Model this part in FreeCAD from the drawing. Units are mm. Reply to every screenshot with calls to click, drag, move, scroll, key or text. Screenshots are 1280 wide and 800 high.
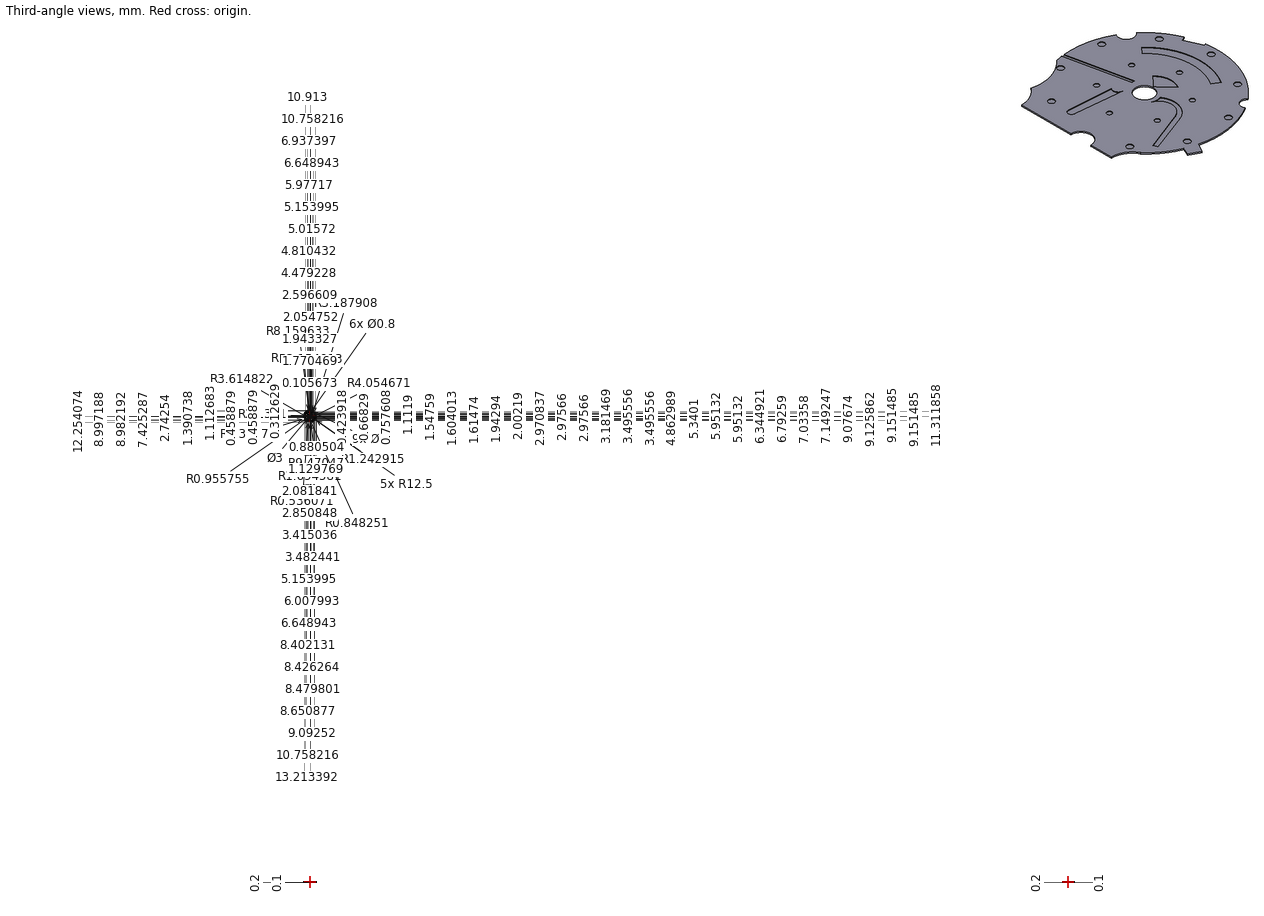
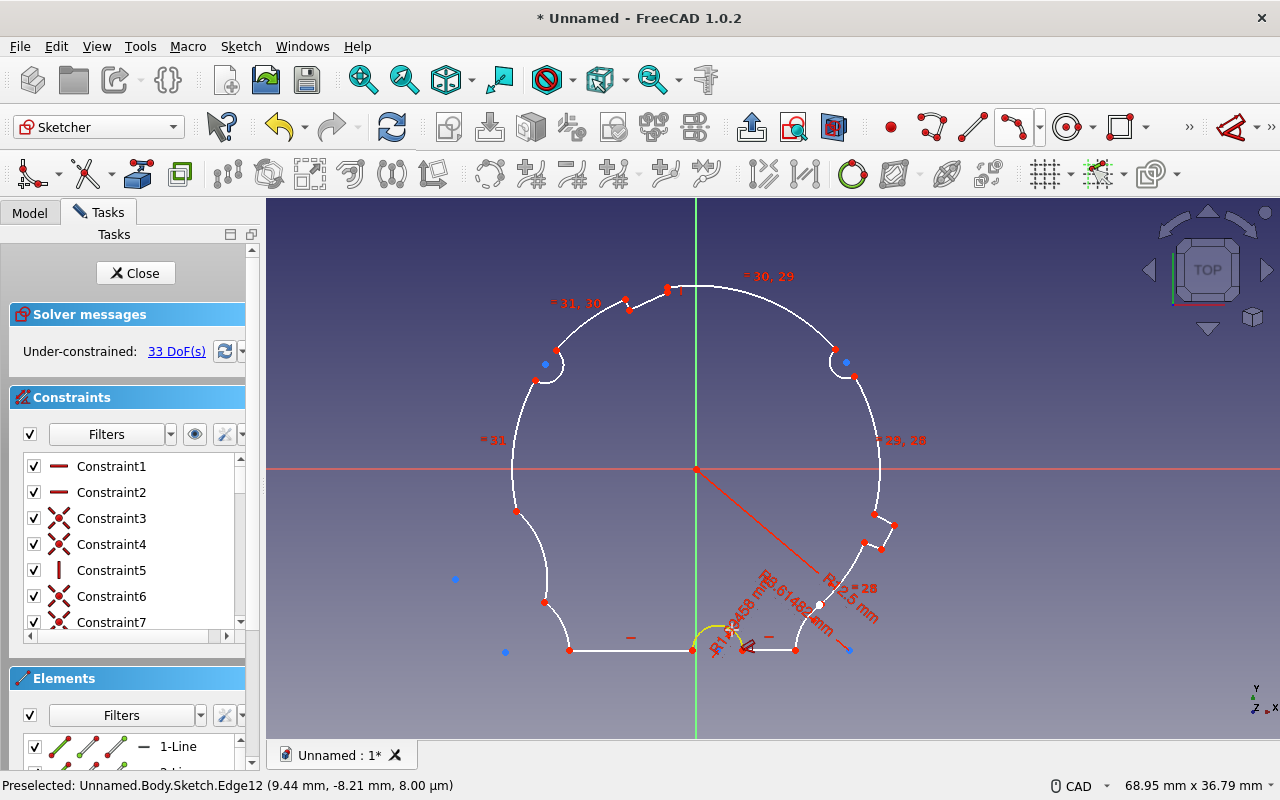
scroll(830, 362, up, 6)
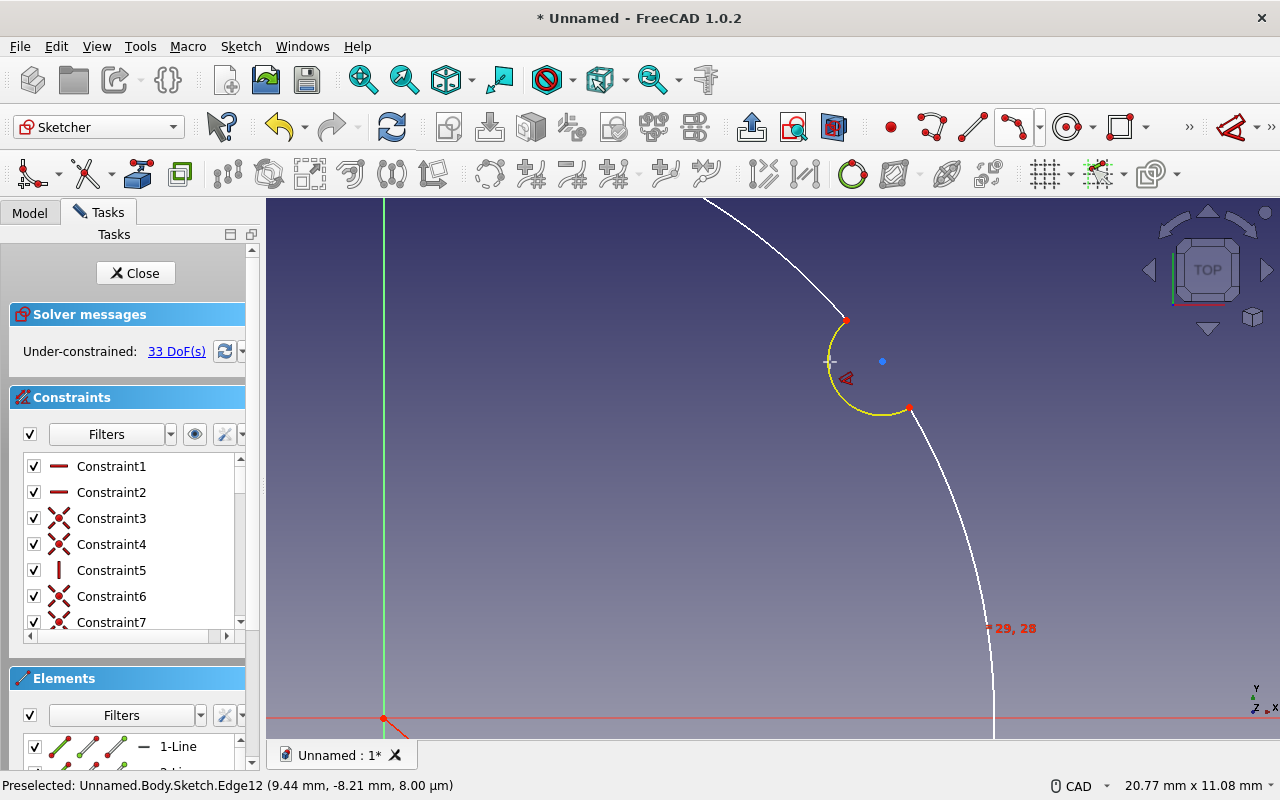
click(828, 363)
click(796, 364)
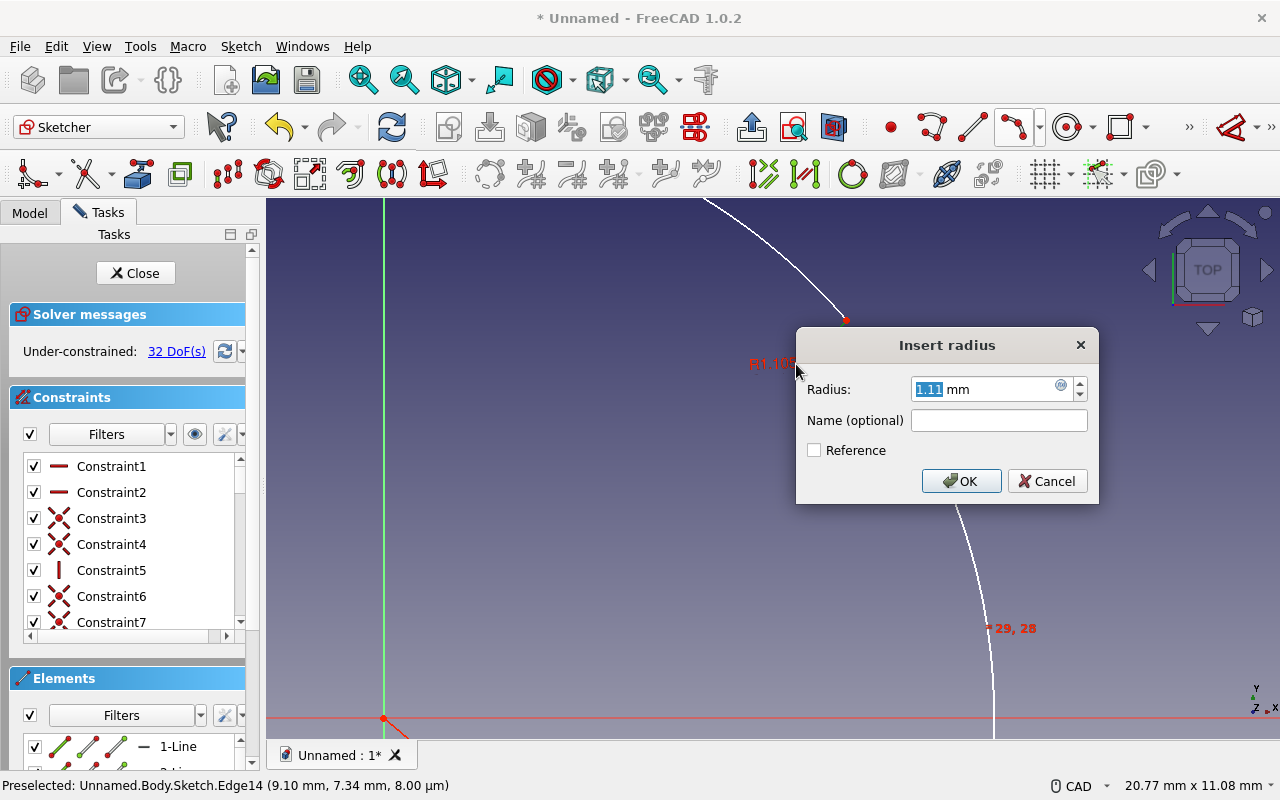
text(0.955755)
key(Return)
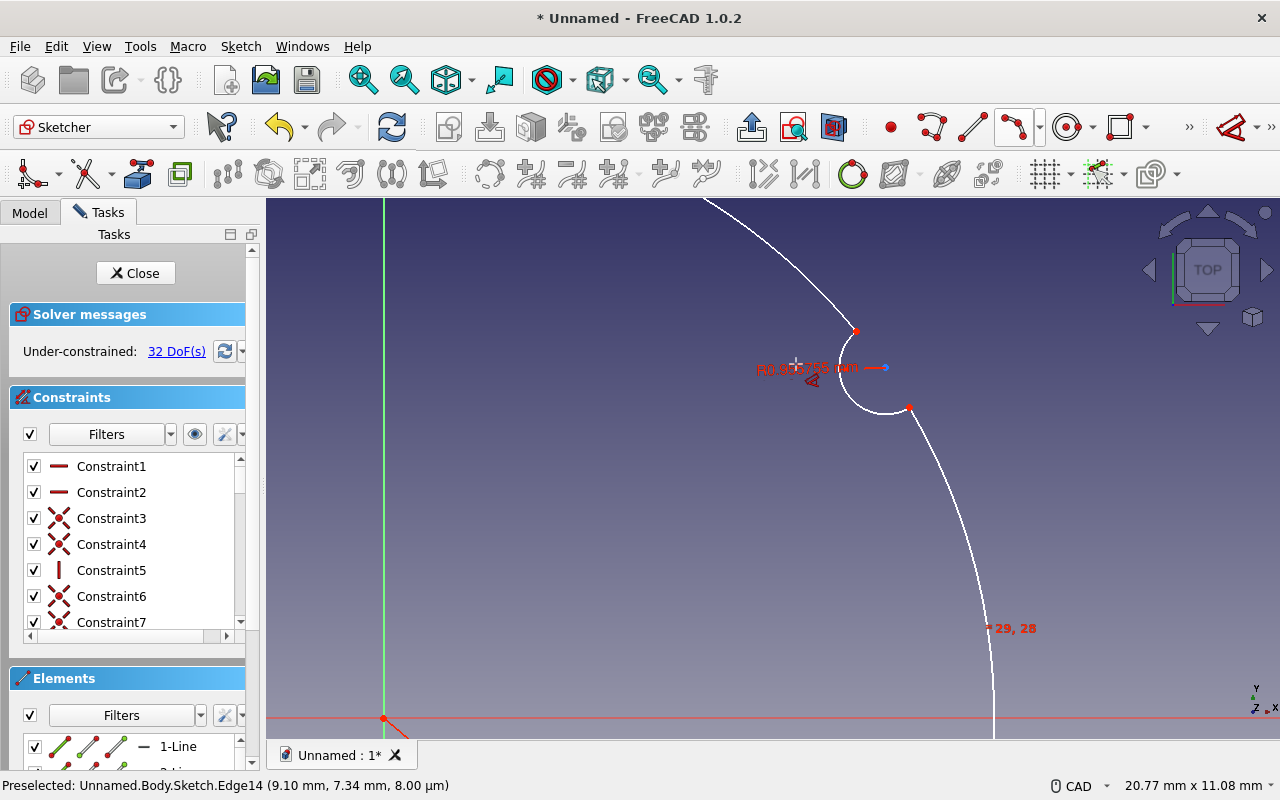
scroll(831, 362, down, 6)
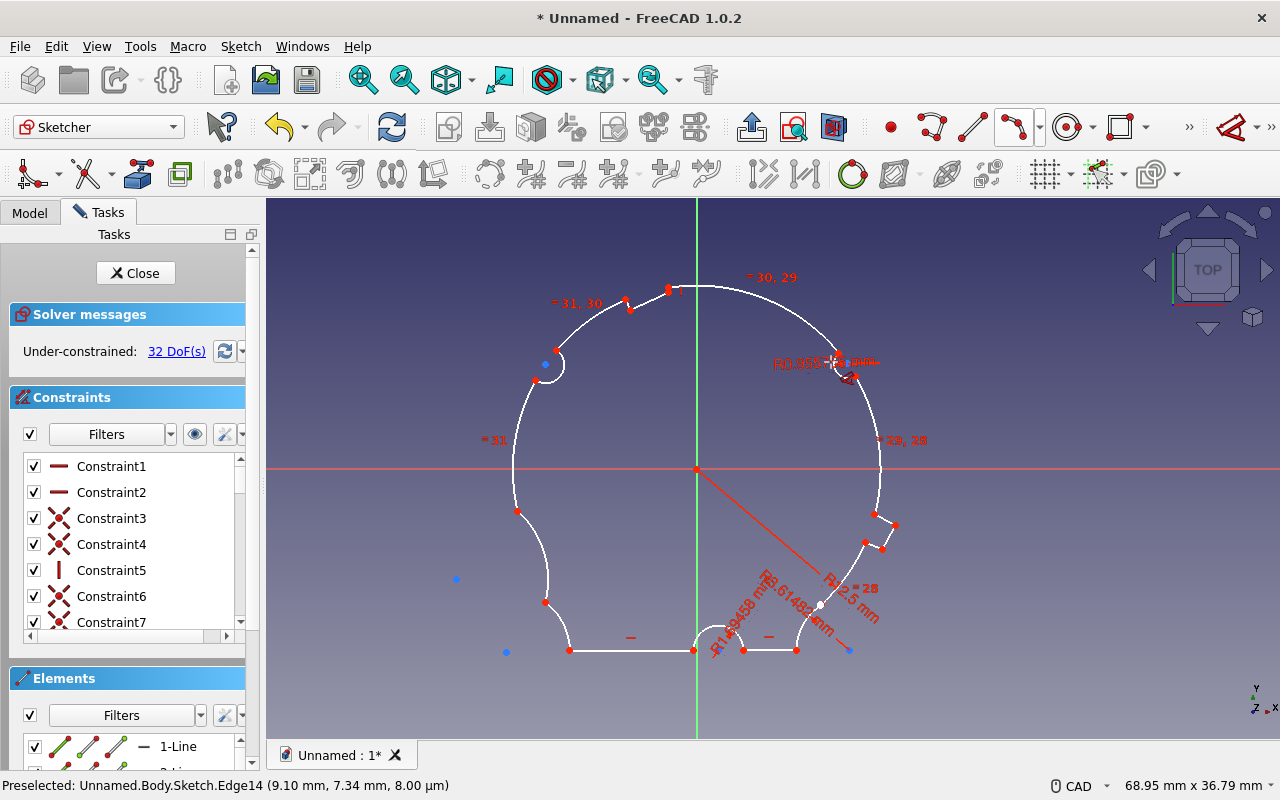
scroll(552, 382, up, 4)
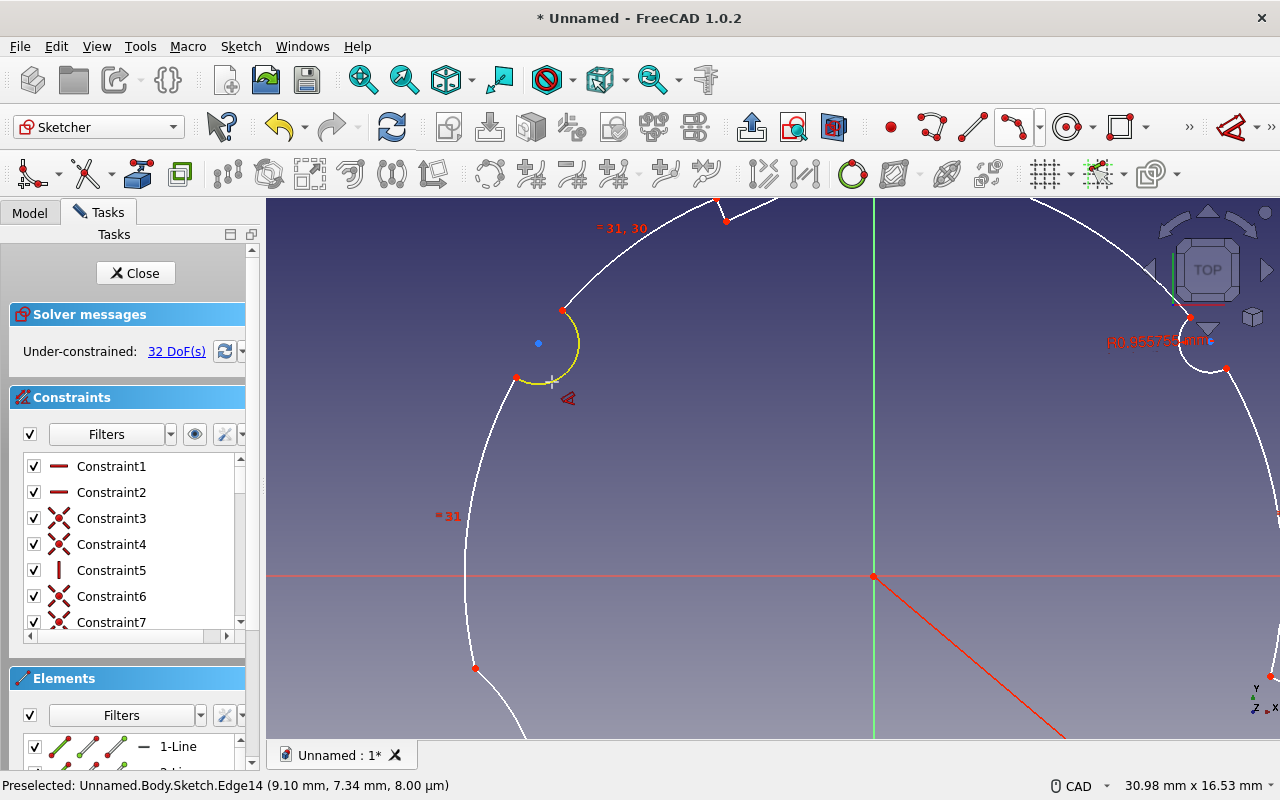
click(552, 382)
click(563, 412)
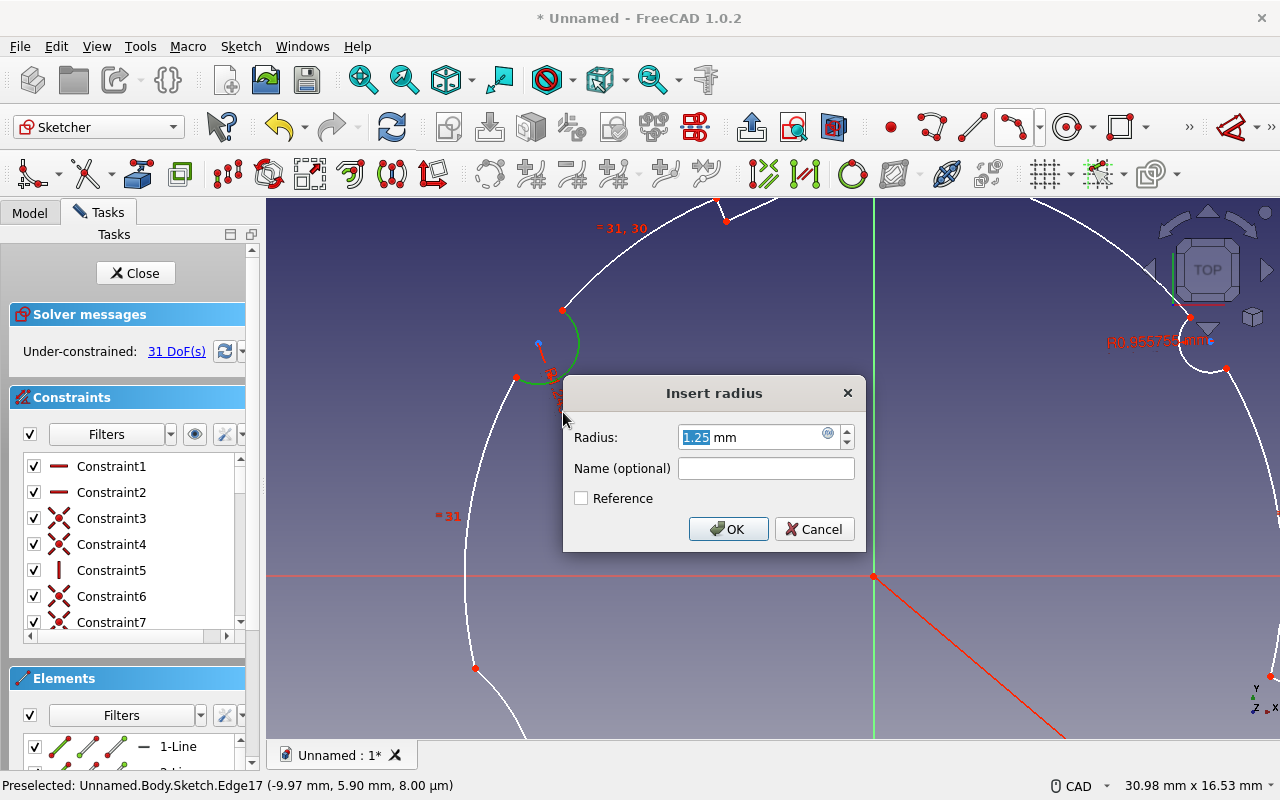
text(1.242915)
key(Return)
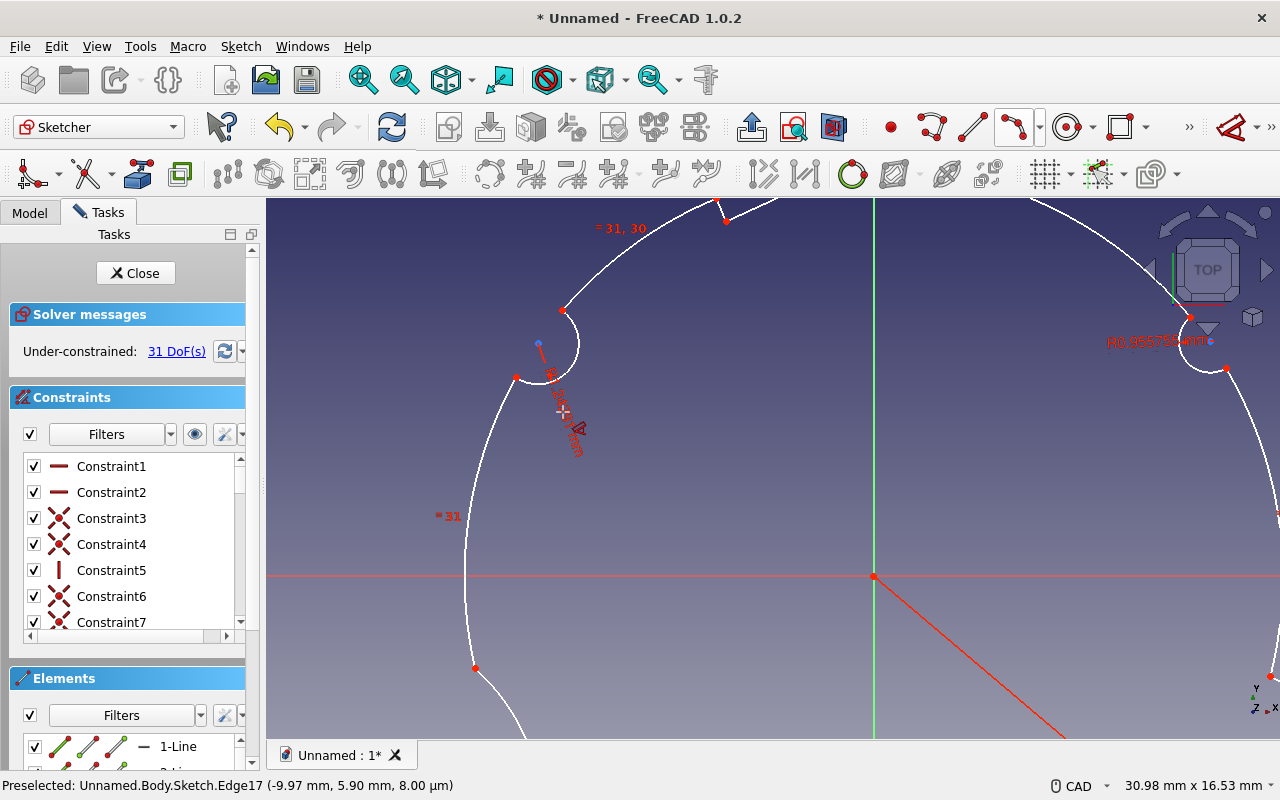
click(505, 702)
click(531, 683)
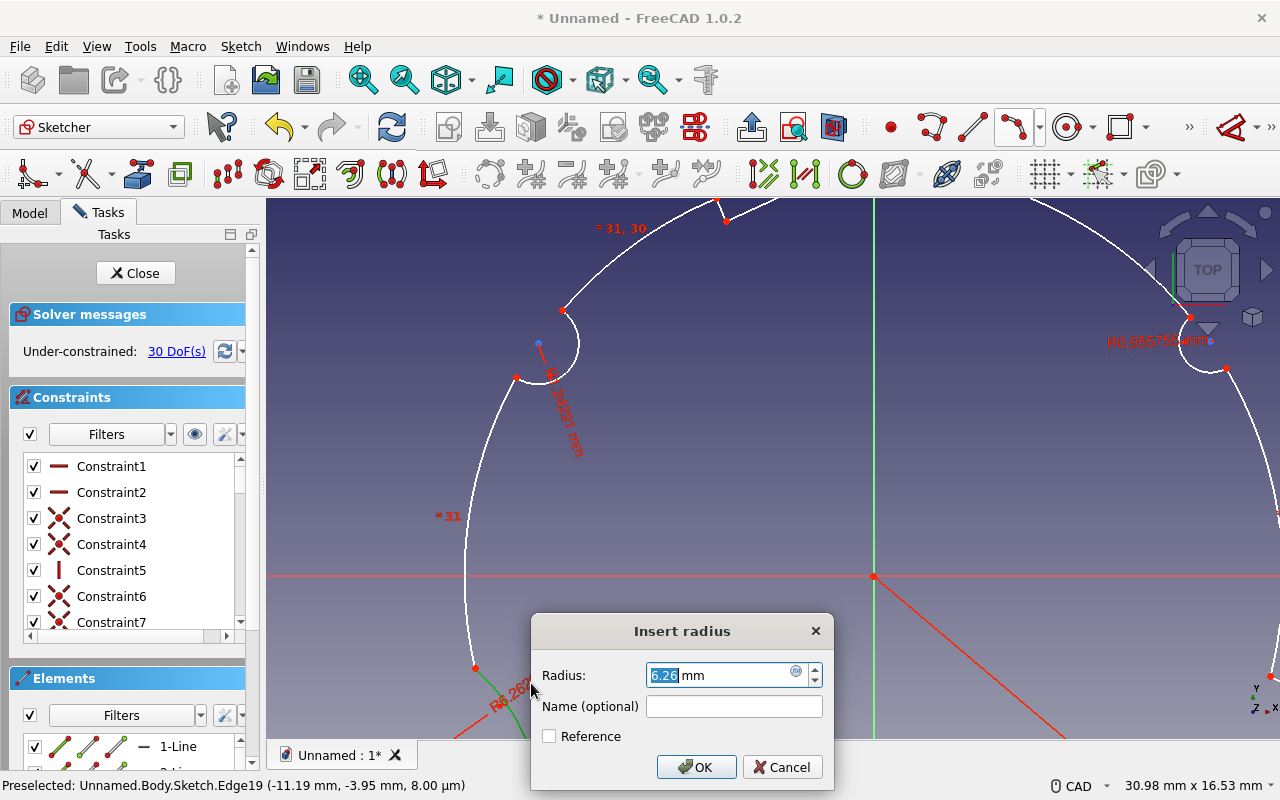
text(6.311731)
key(Return)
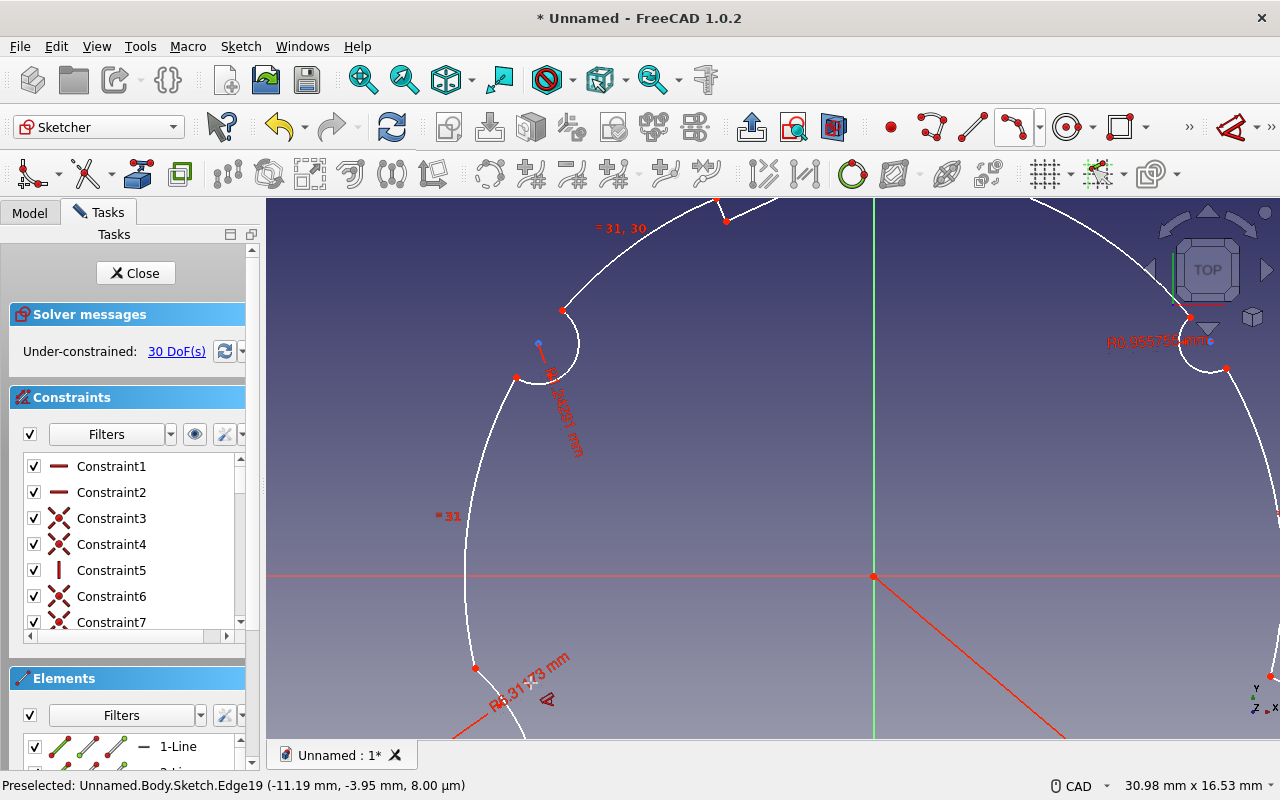
scroll(551, 382, down, 4)